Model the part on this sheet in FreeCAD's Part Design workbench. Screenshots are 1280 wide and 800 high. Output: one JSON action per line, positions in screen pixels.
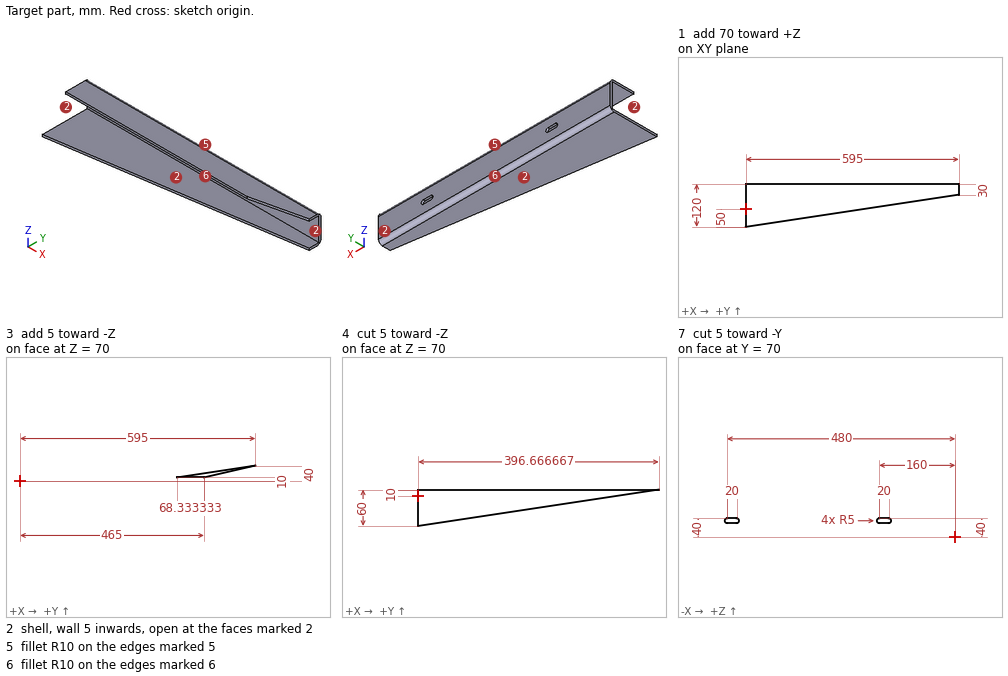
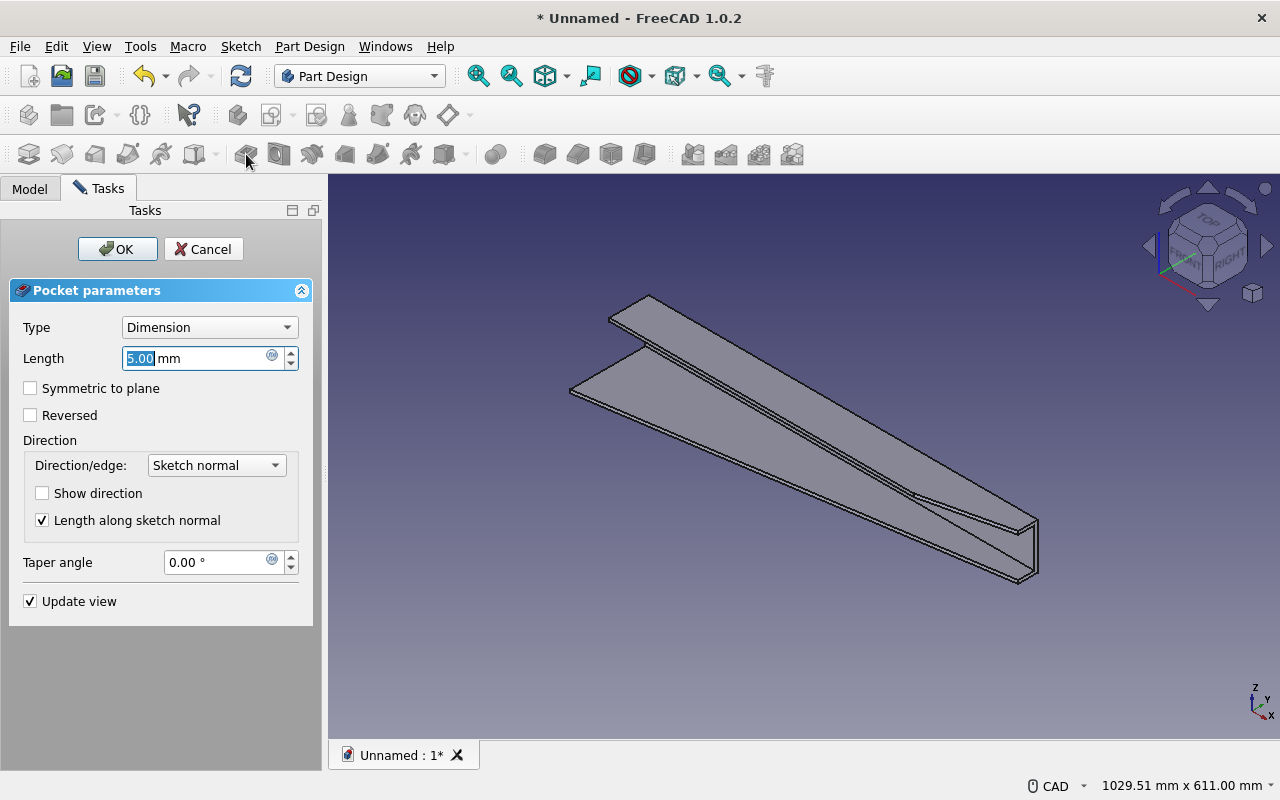
{"action": "type", "text": "5"}
{"action": "key", "text": "Tab"}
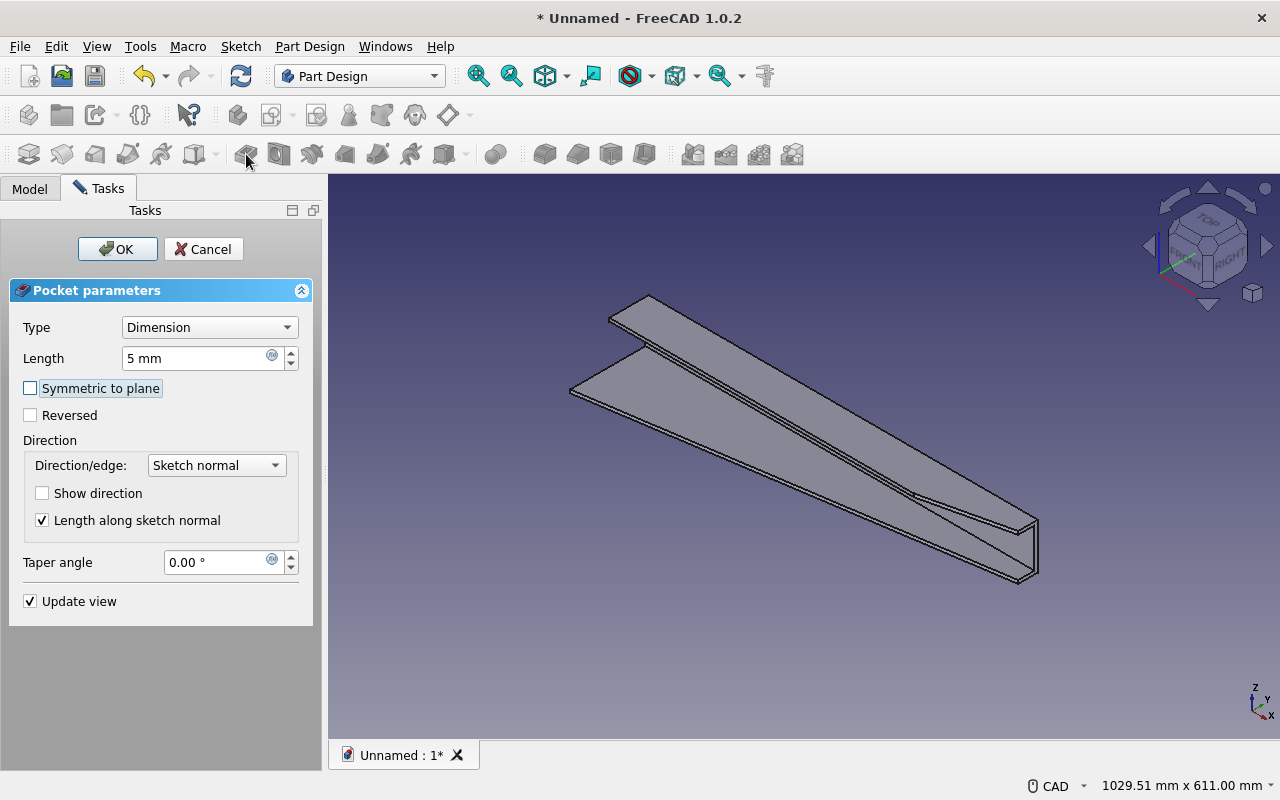
{"action": "left_click", "coordinate": [118, 249]}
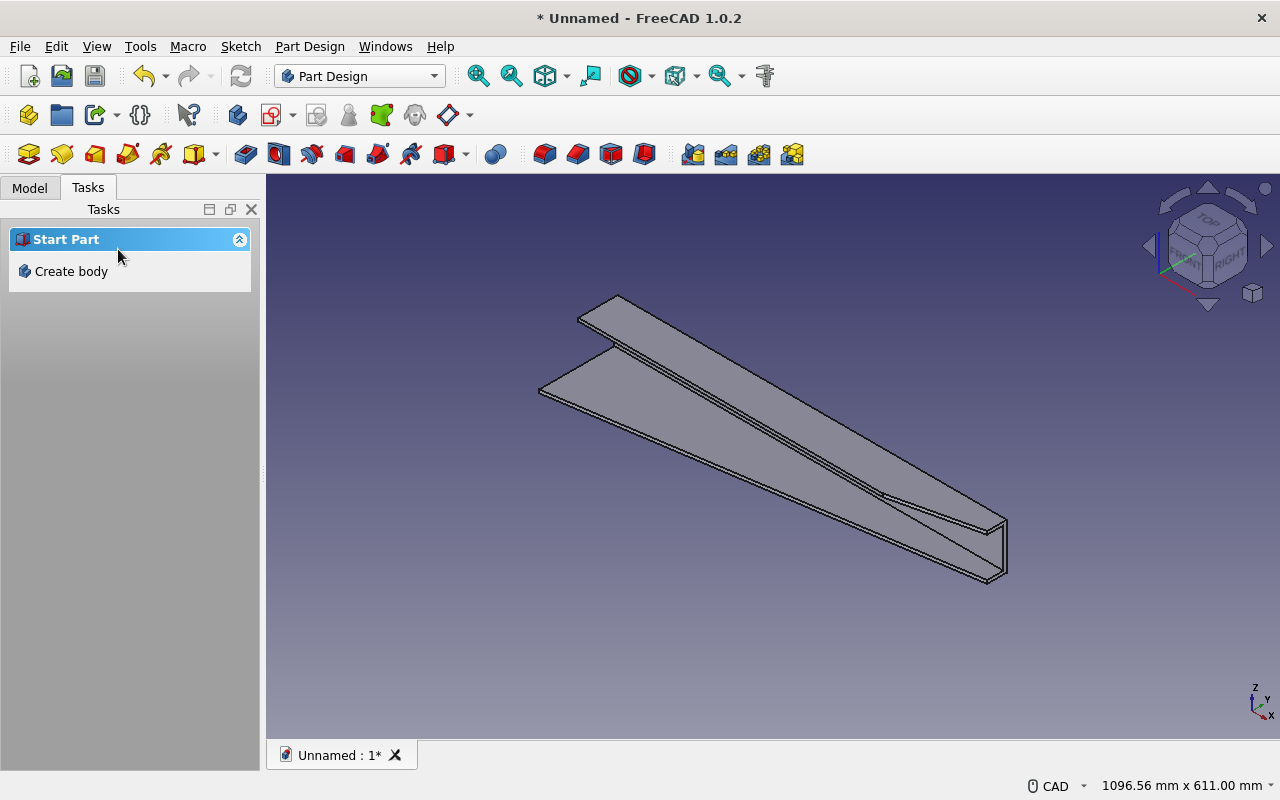
{"action": "key", "text": "2"}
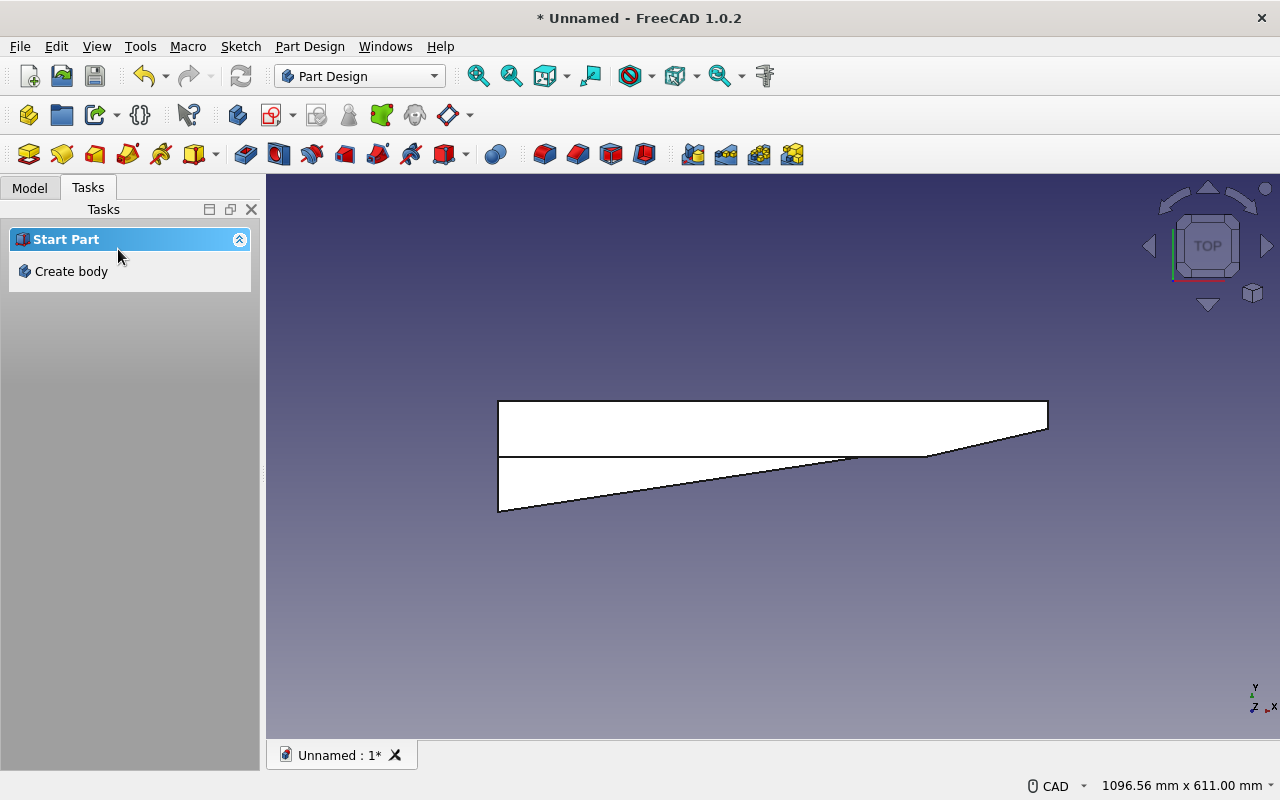
{"action": "left_click", "coordinate": [773, 400]}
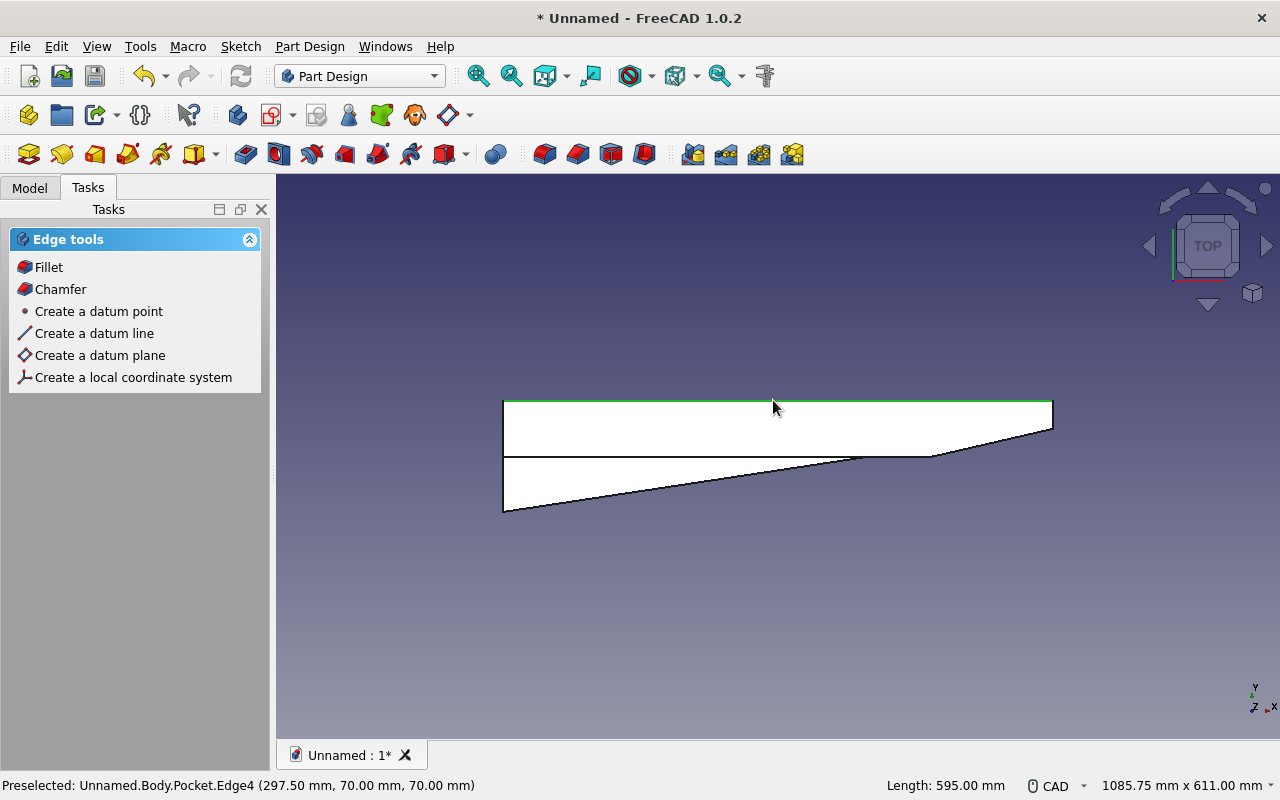
{"action": "left_click", "coordinate": [545, 154]}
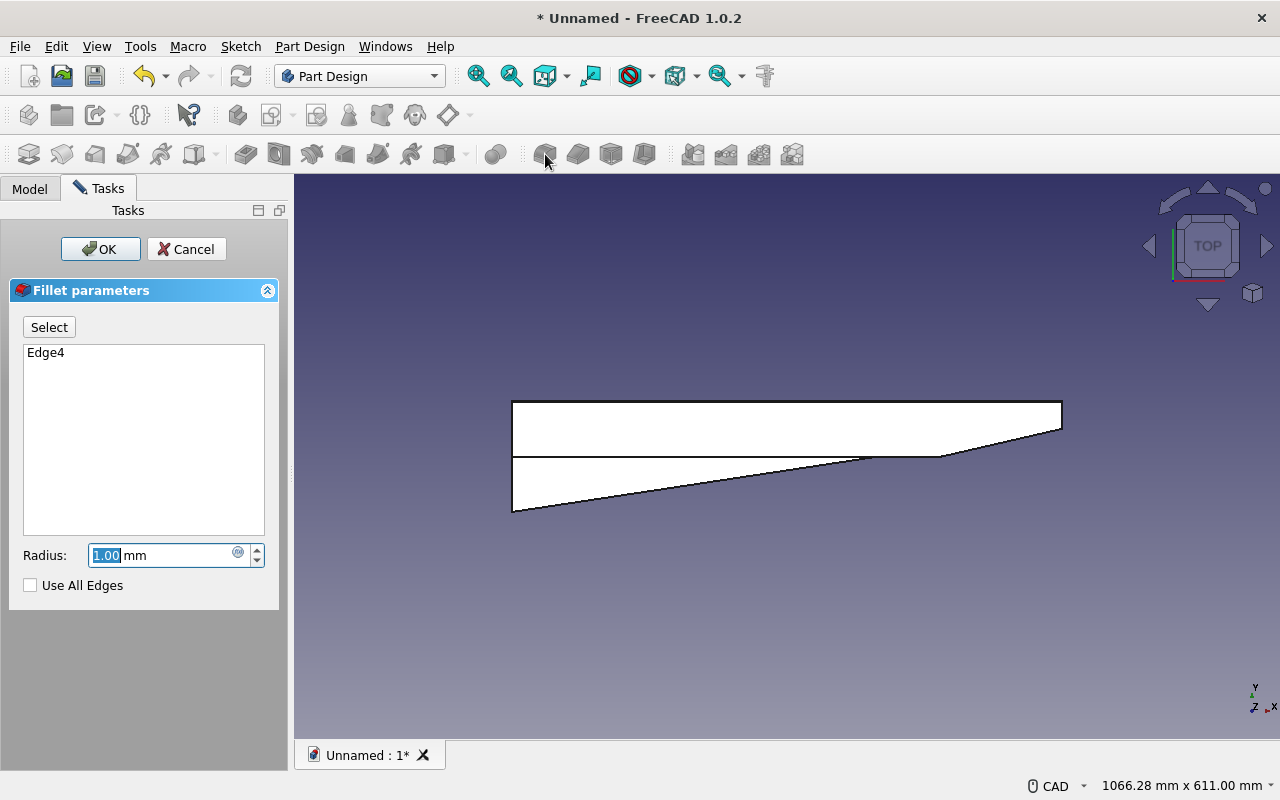
{"action": "type", "text": "10"}
{"action": "key", "text": "Tab"}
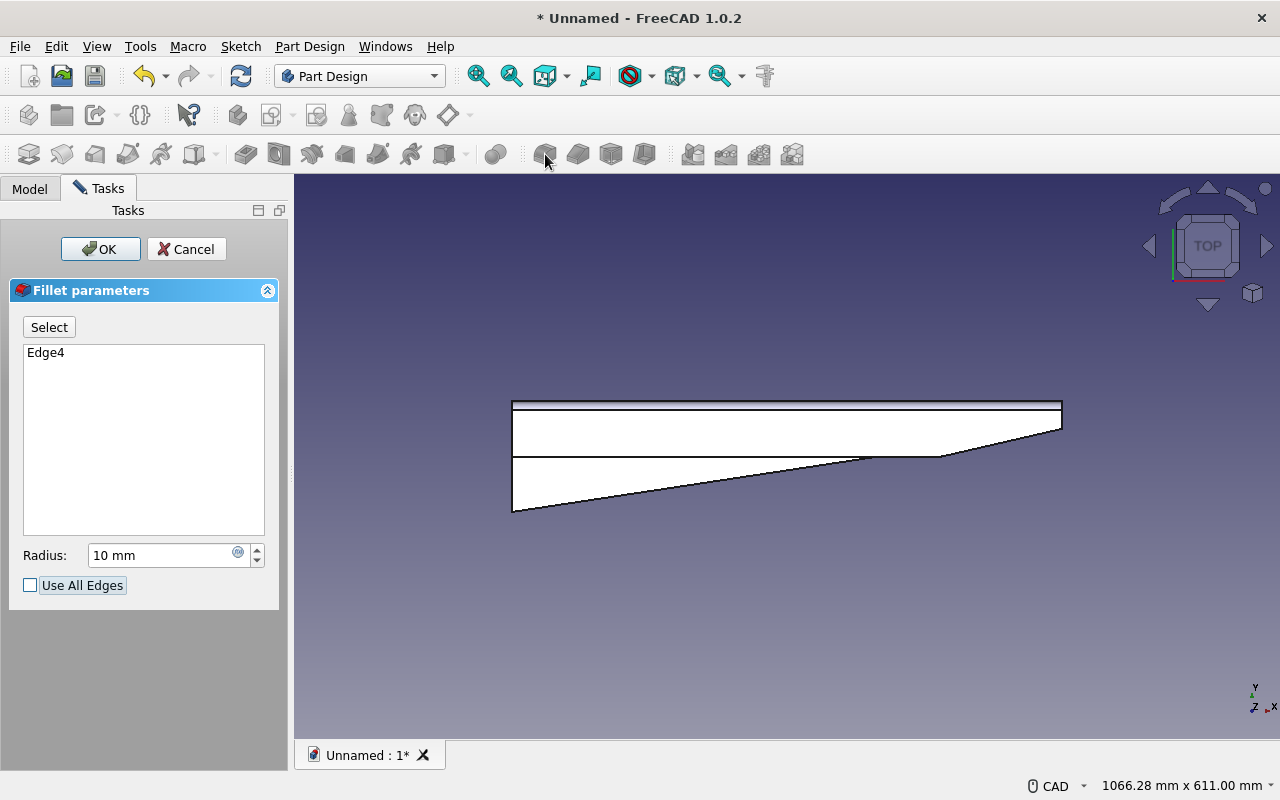
{"action": "left_click", "coordinate": [101, 249]}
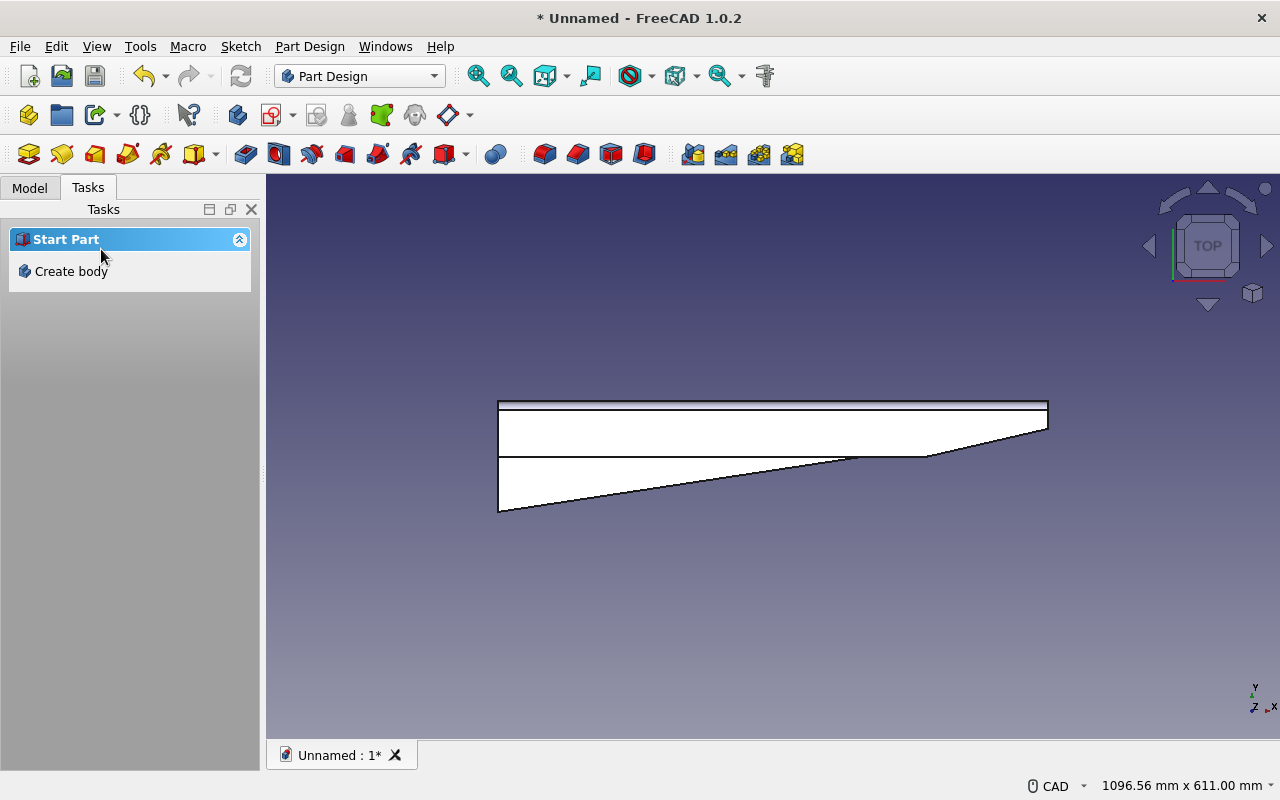
{"action": "key", "text": "0"}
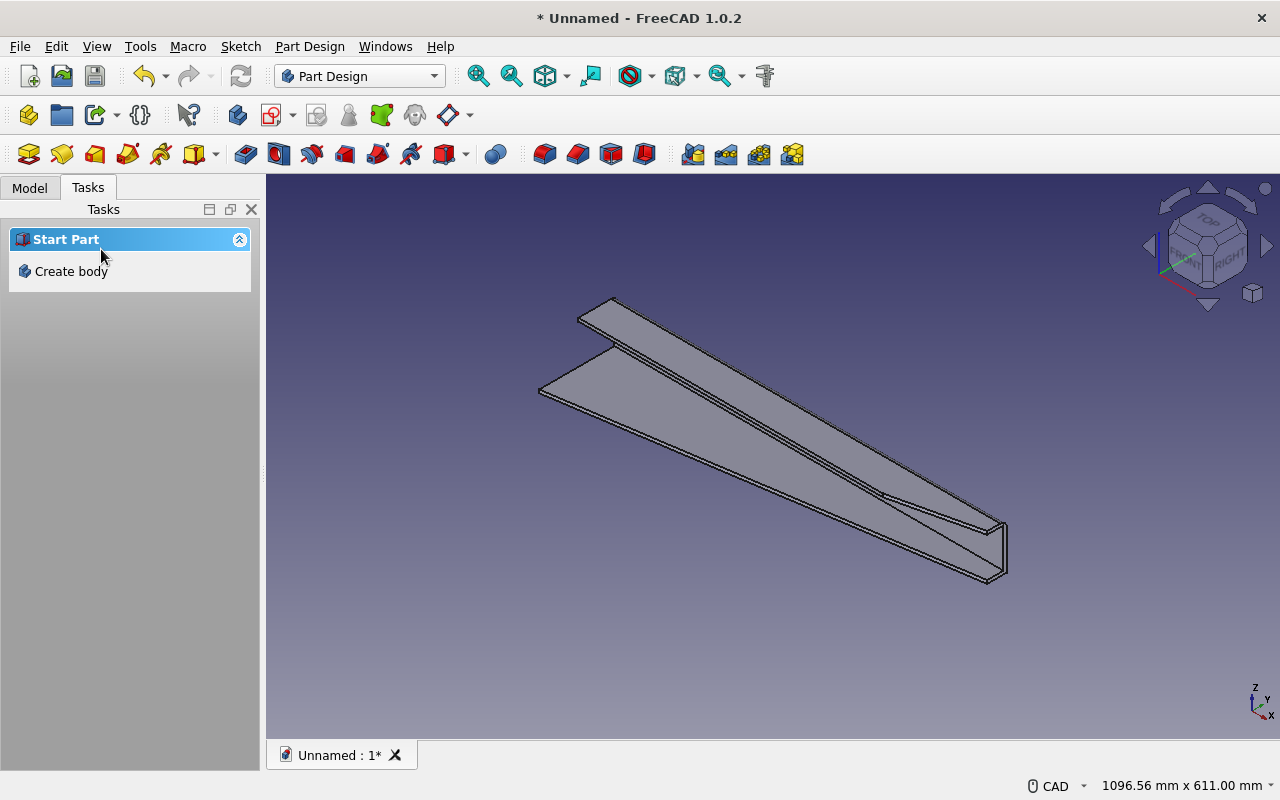
{"action": "key", "text": "2"}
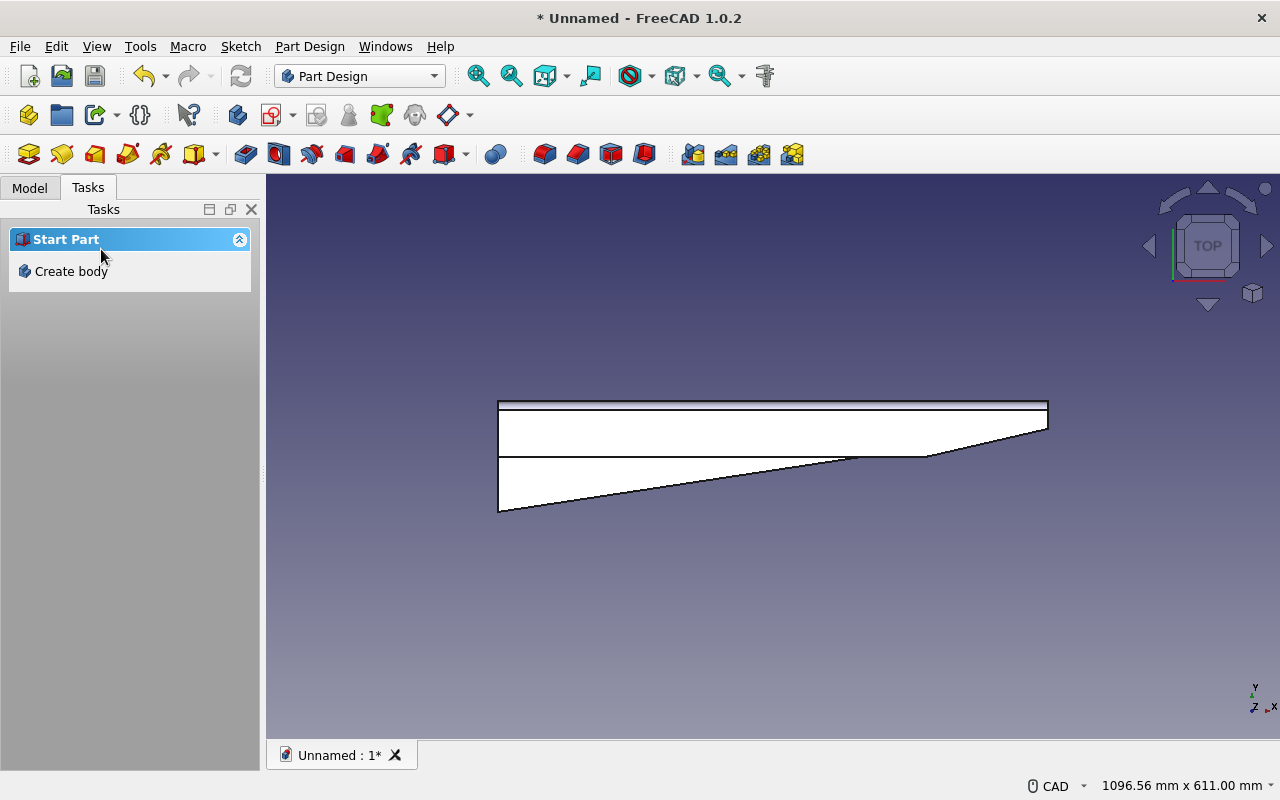
{"action": "key", "text": "1"}